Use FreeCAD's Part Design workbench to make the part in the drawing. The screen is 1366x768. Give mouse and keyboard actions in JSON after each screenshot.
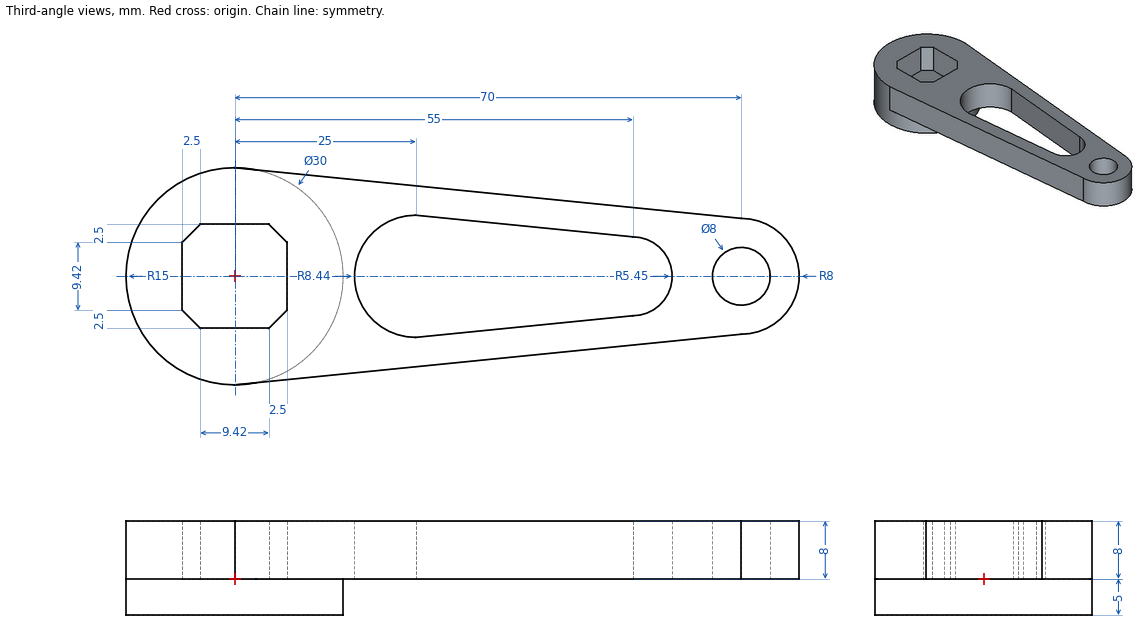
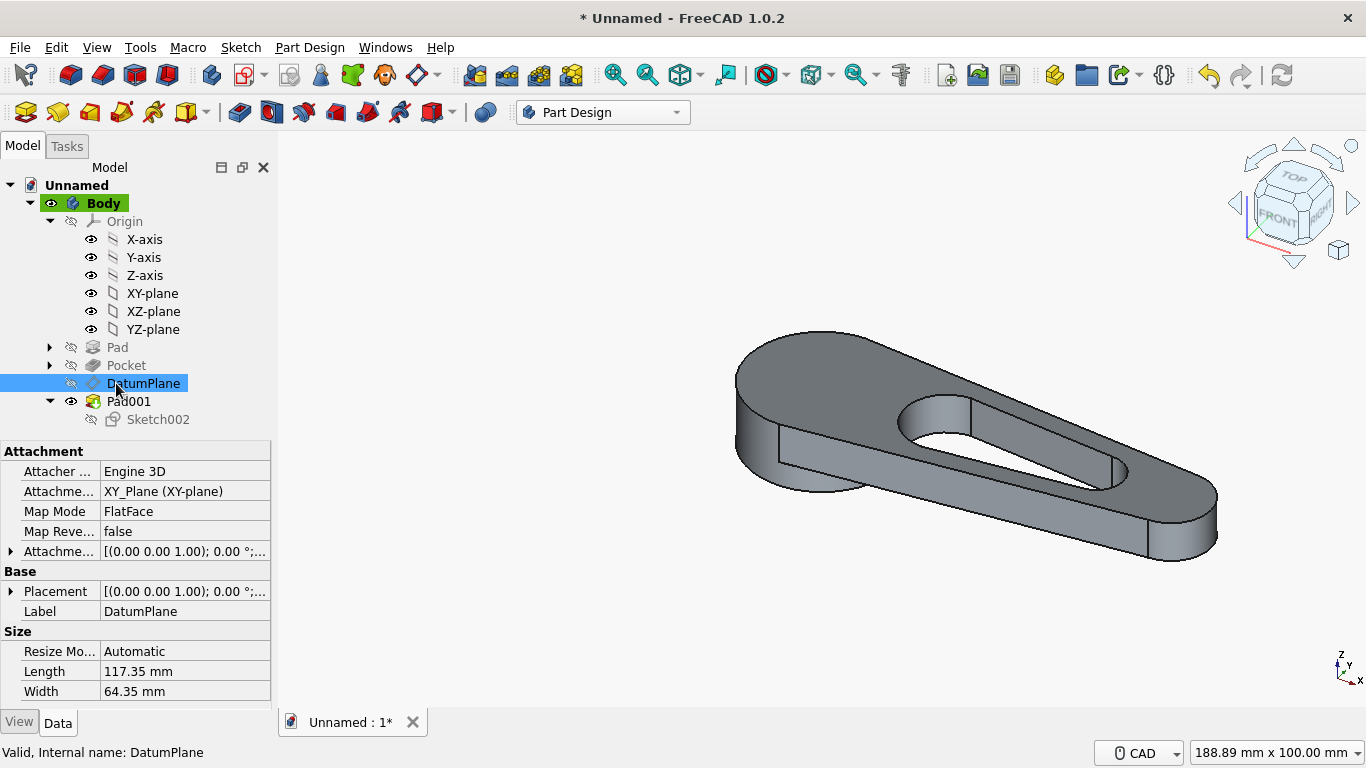
{"action": "left_click", "coordinate": [847, 388]}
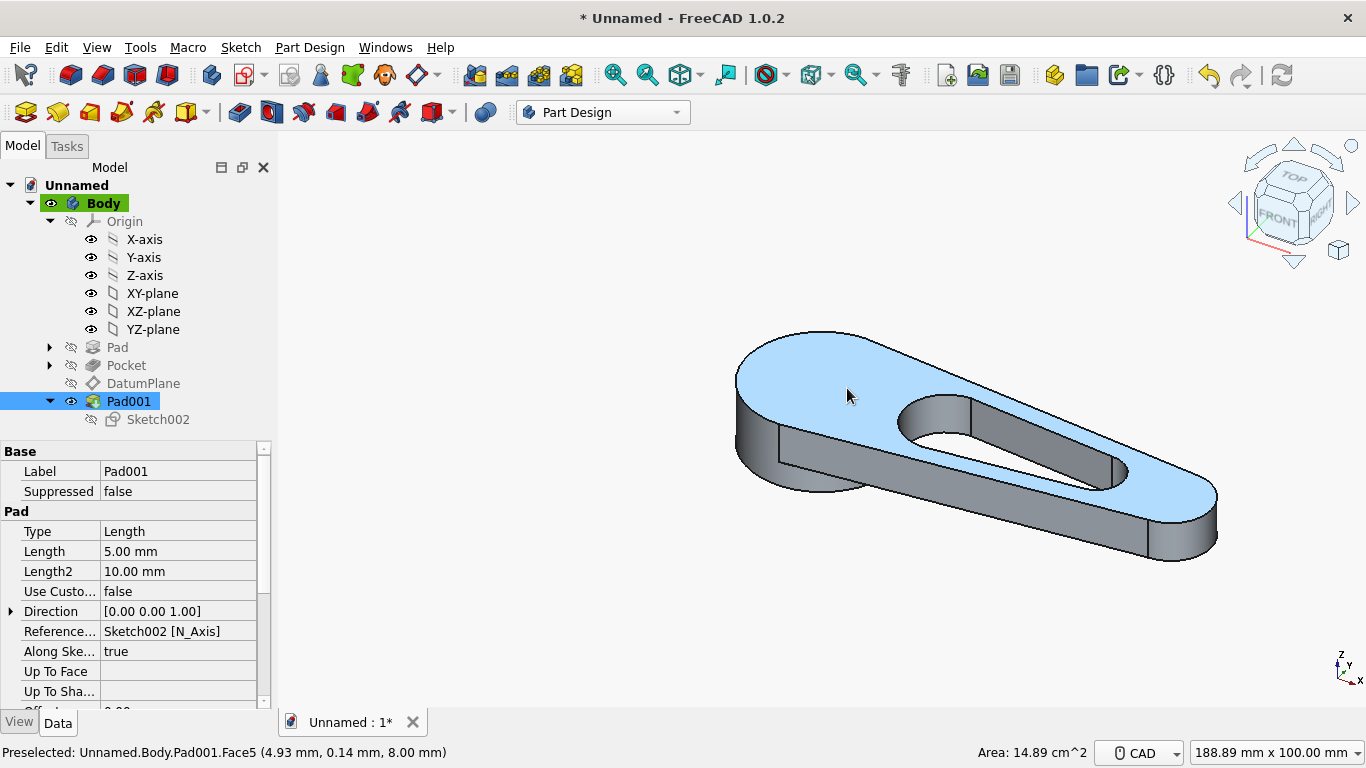
{"action": "left_click", "coordinate": [244, 76]}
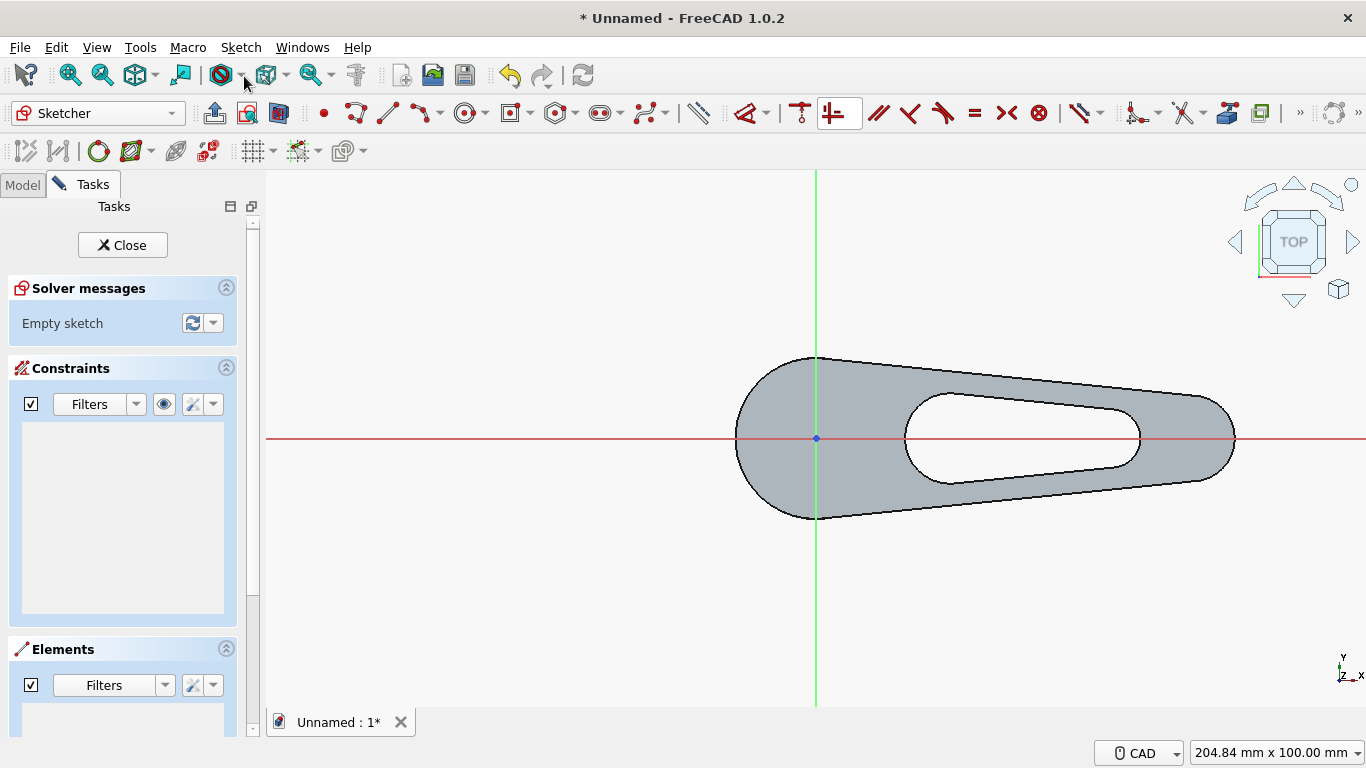
{"action": "scroll", "coordinate": [748, 438], "scroll_direction": "down", "scroll_amount": 5}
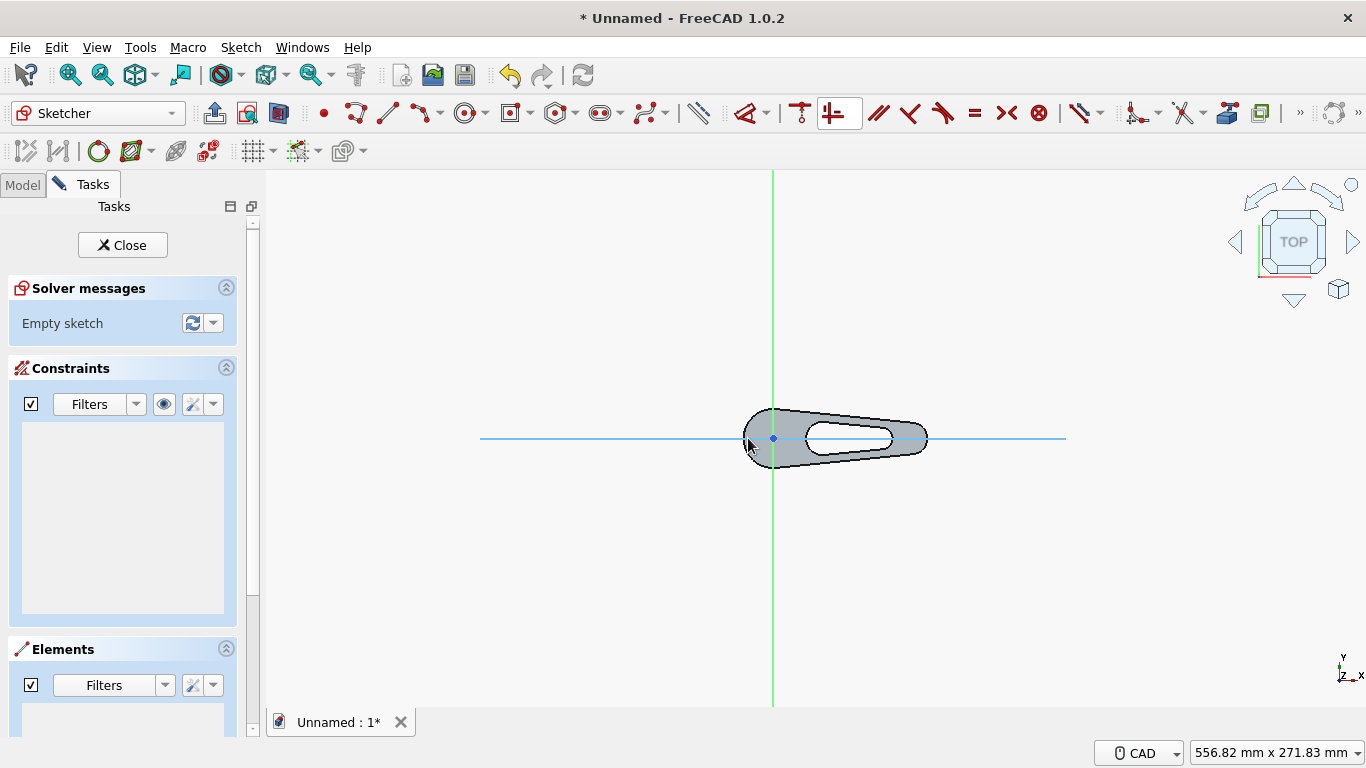
{"action": "scroll", "coordinate": [920, 438], "scroll_direction": "up", "scroll_amount": 15}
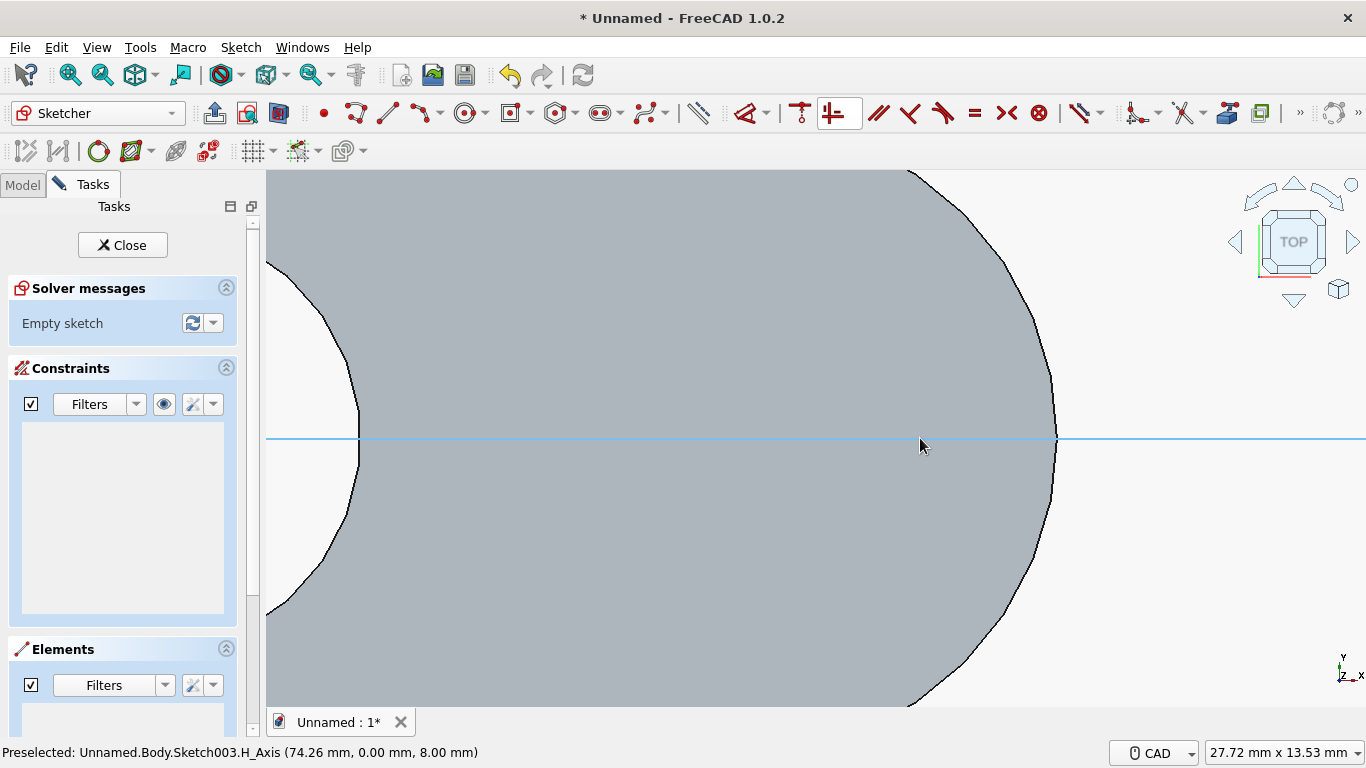
{"action": "left_click", "coordinate": [466, 114]}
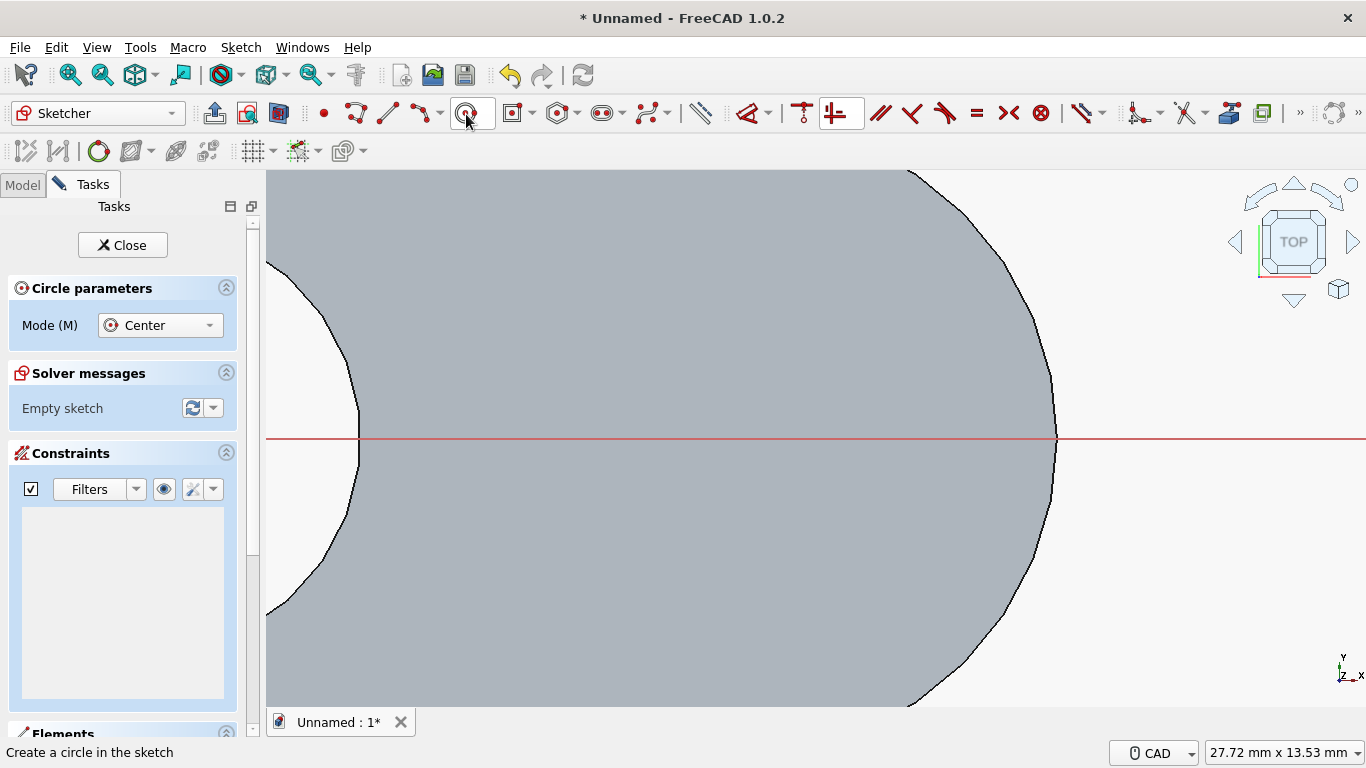
{"action": "left_click", "coordinate": [740, 438]}
{"action": "left_click", "coordinate": [852, 326]}
{"action": "key", "text": "Escape"}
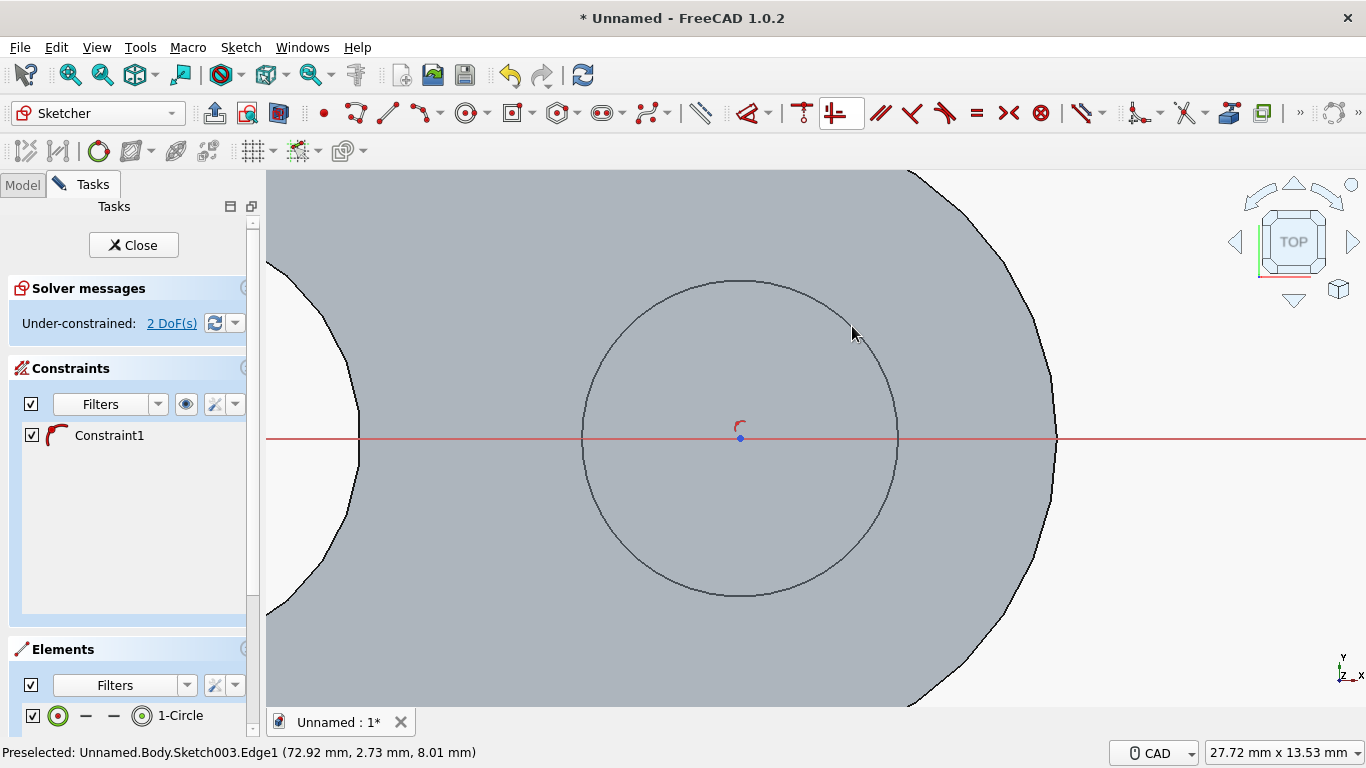
{"action": "left_click", "coordinate": [748, 114]}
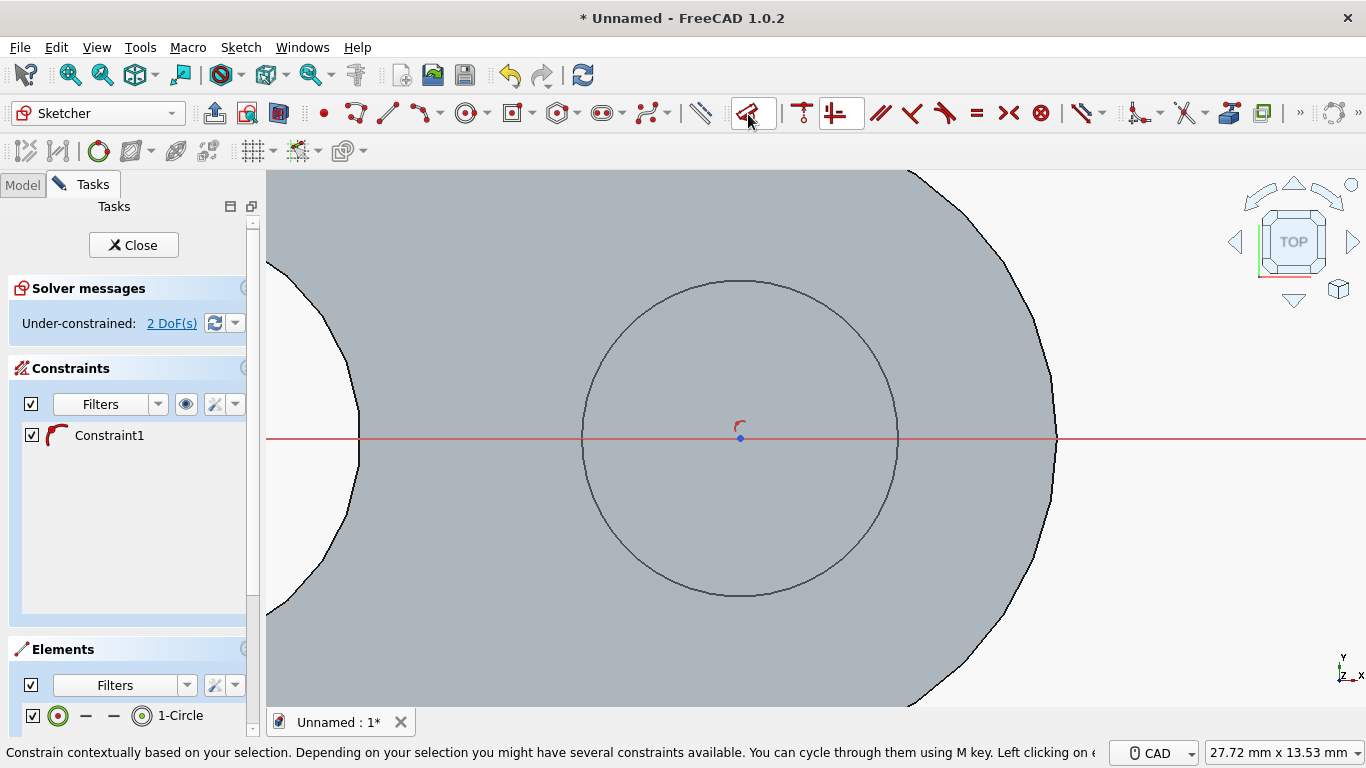
{"action": "left_click", "coordinate": [851, 326]}
{"action": "left_click", "coordinate": [873, 303]}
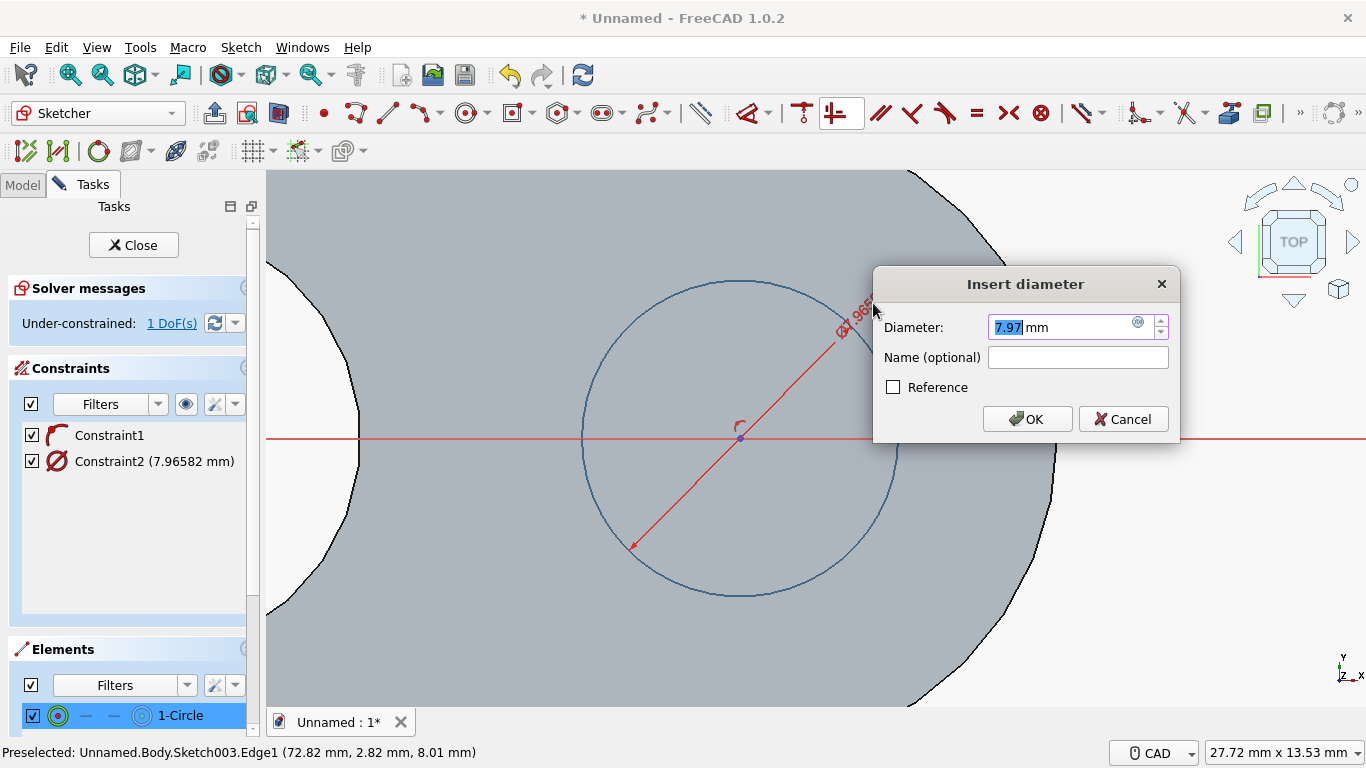
{"action": "type", "text": "8"}
{"action": "key", "text": "Return"}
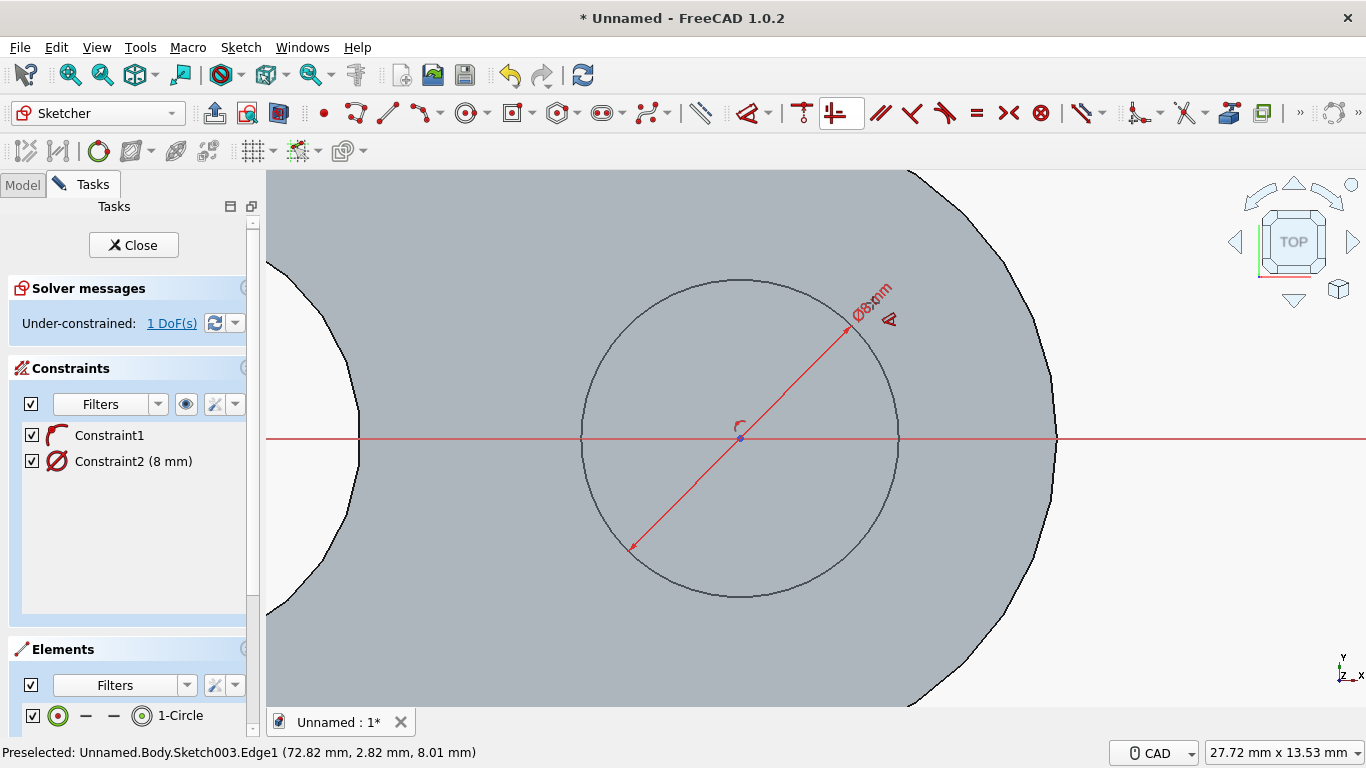
{"action": "left_click", "coordinate": [740, 438]}
{"action": "left_click", "coordinate": [517, 472]}